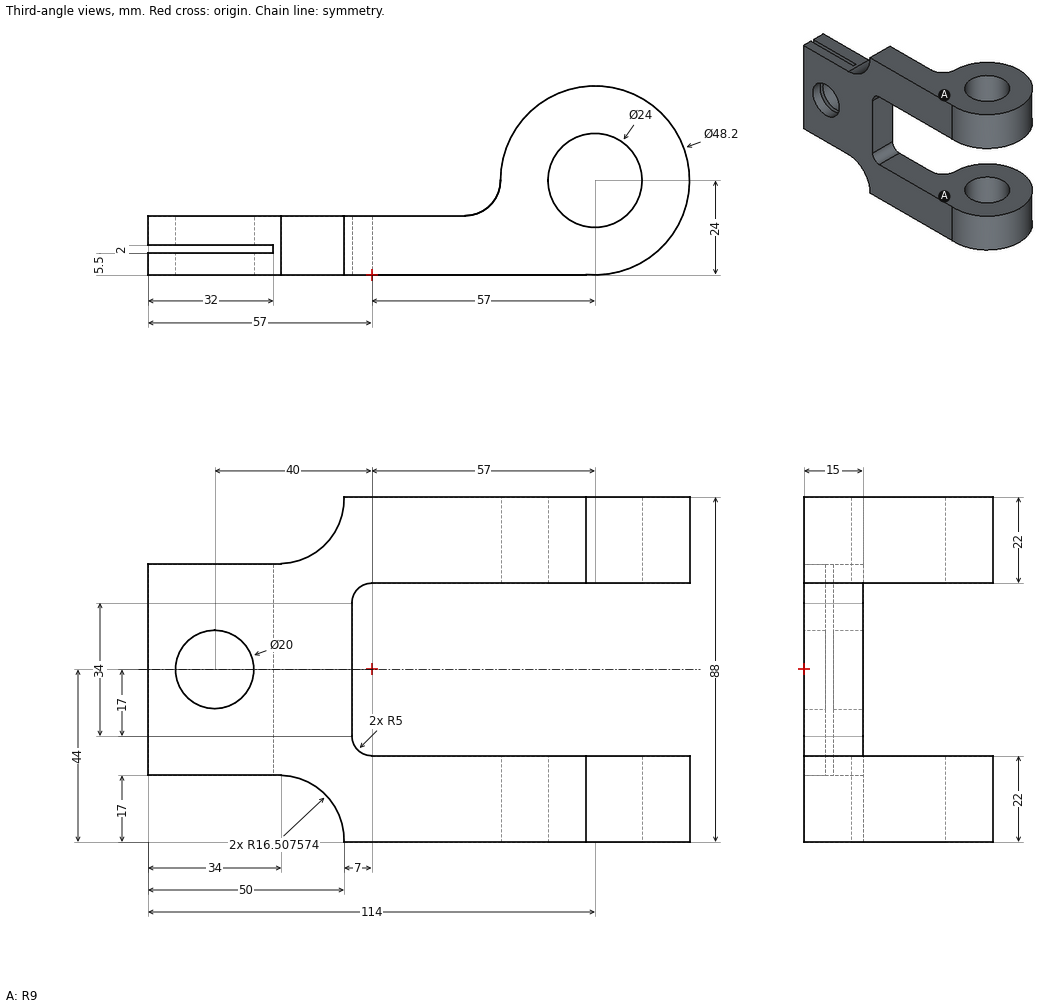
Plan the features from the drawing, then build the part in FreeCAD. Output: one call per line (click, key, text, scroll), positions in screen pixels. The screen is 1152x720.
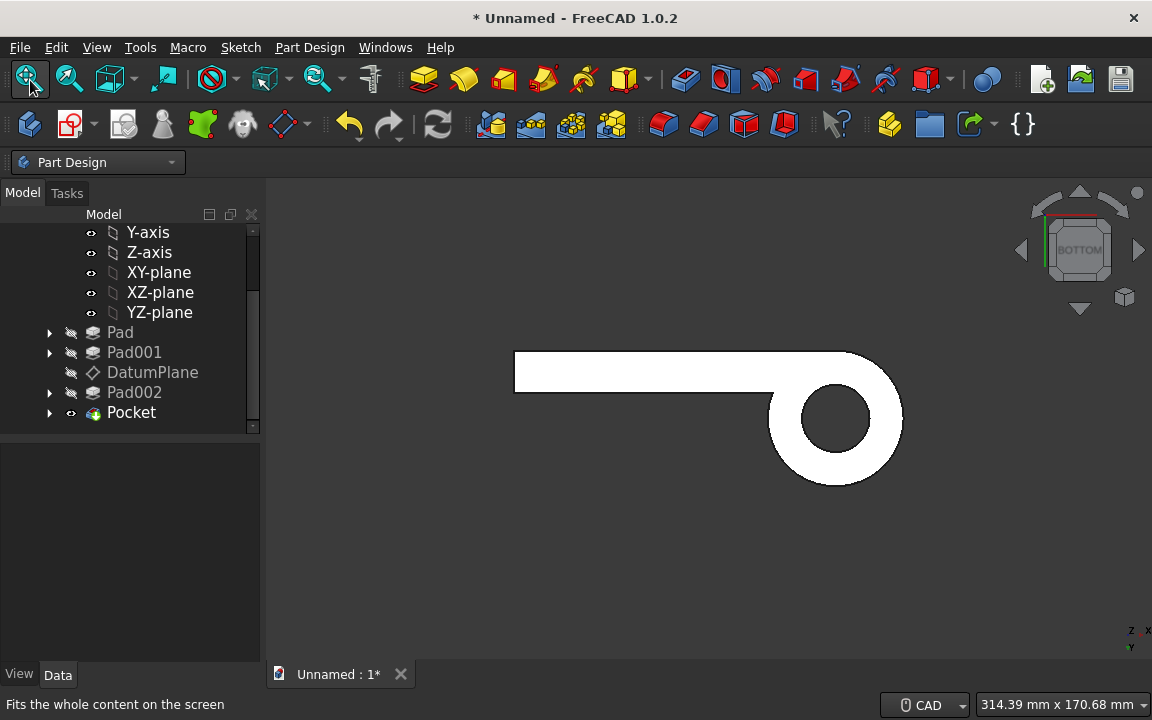
key(4)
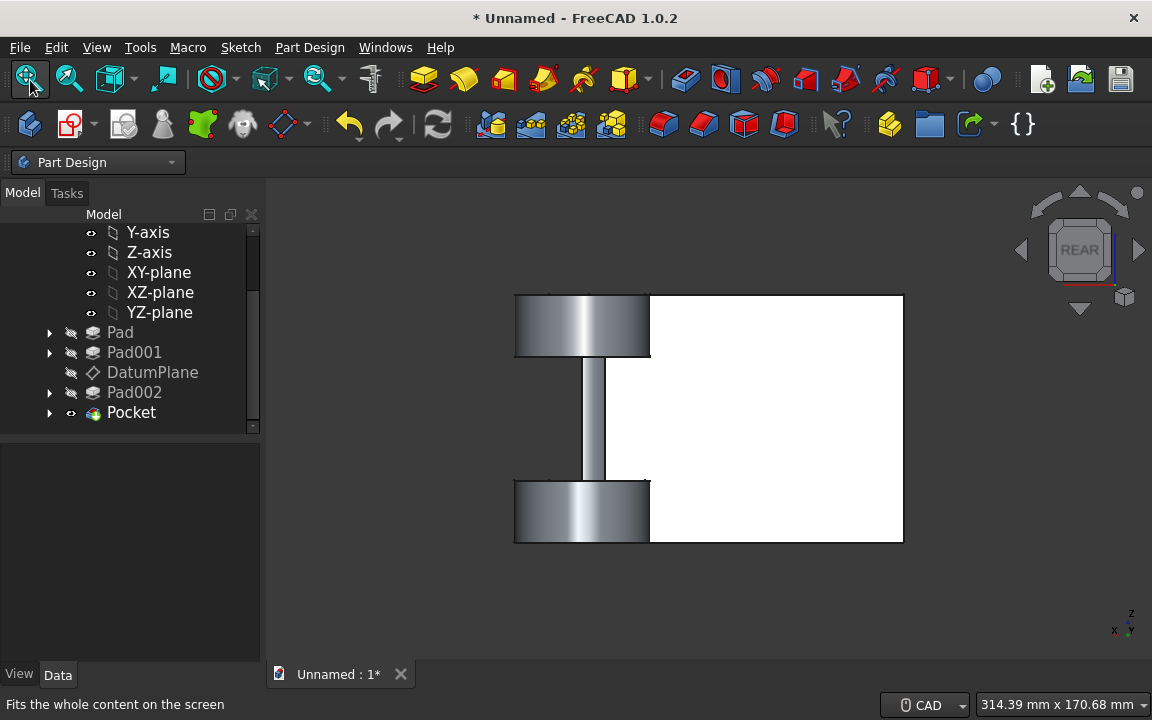
key(6)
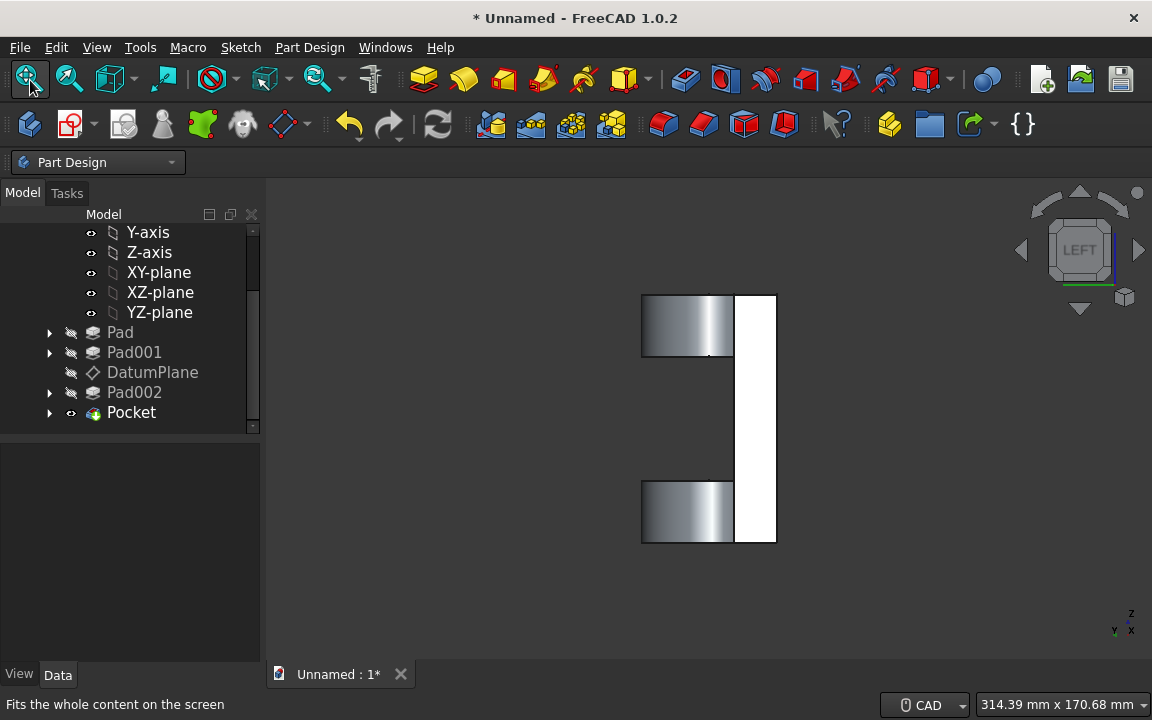
key(v)
key(3)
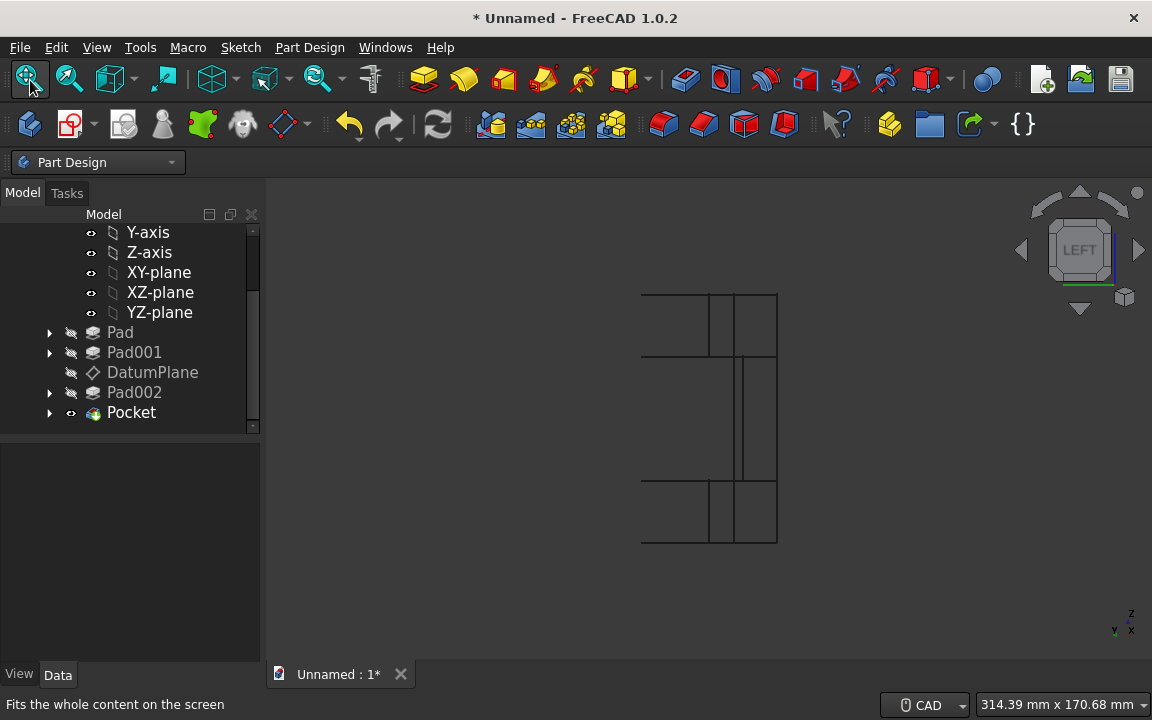
key(0)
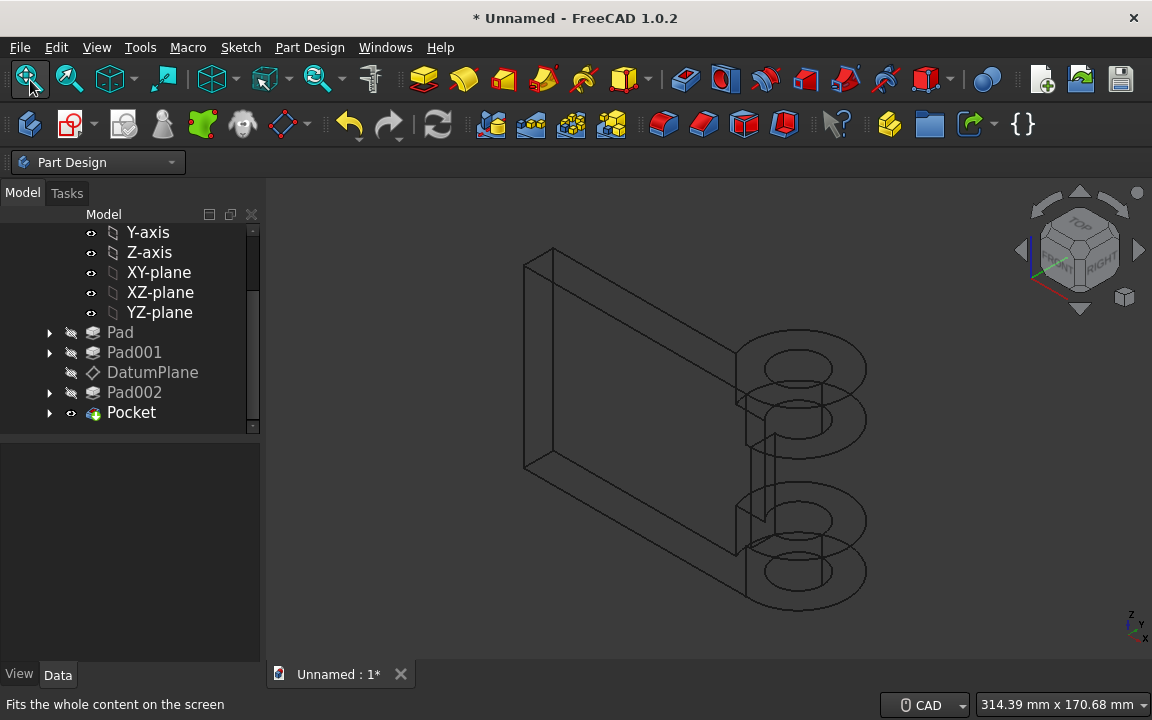
click(736, 378)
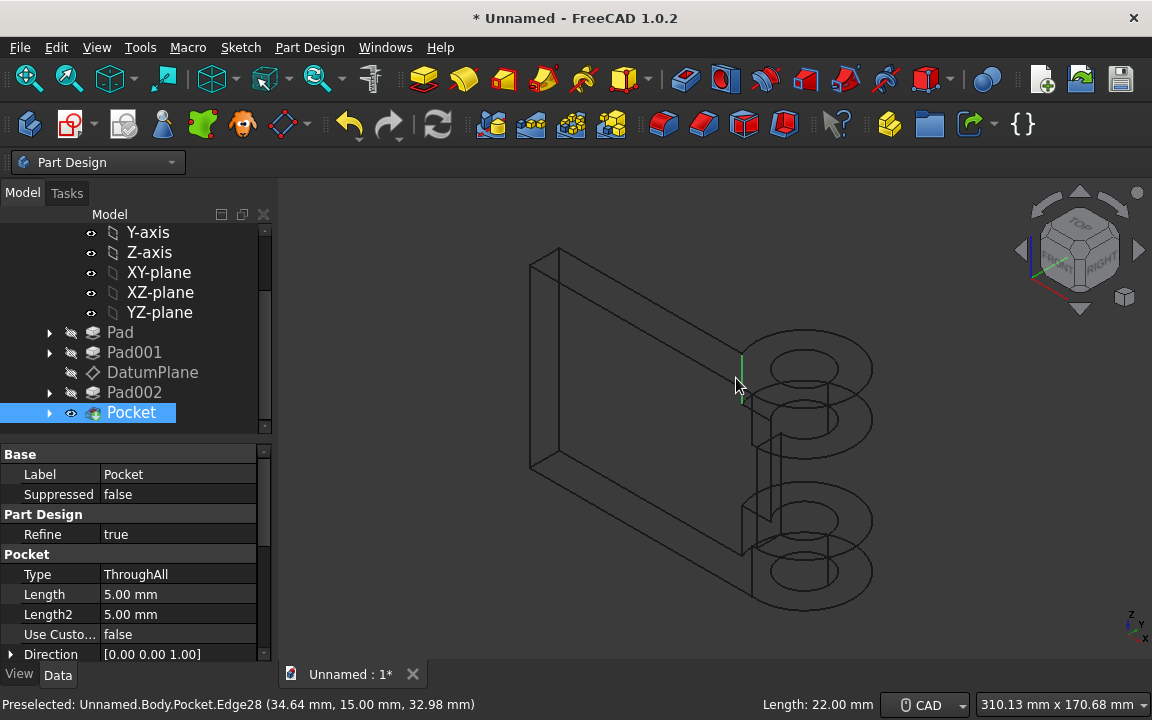
click(742, 530, ctrl)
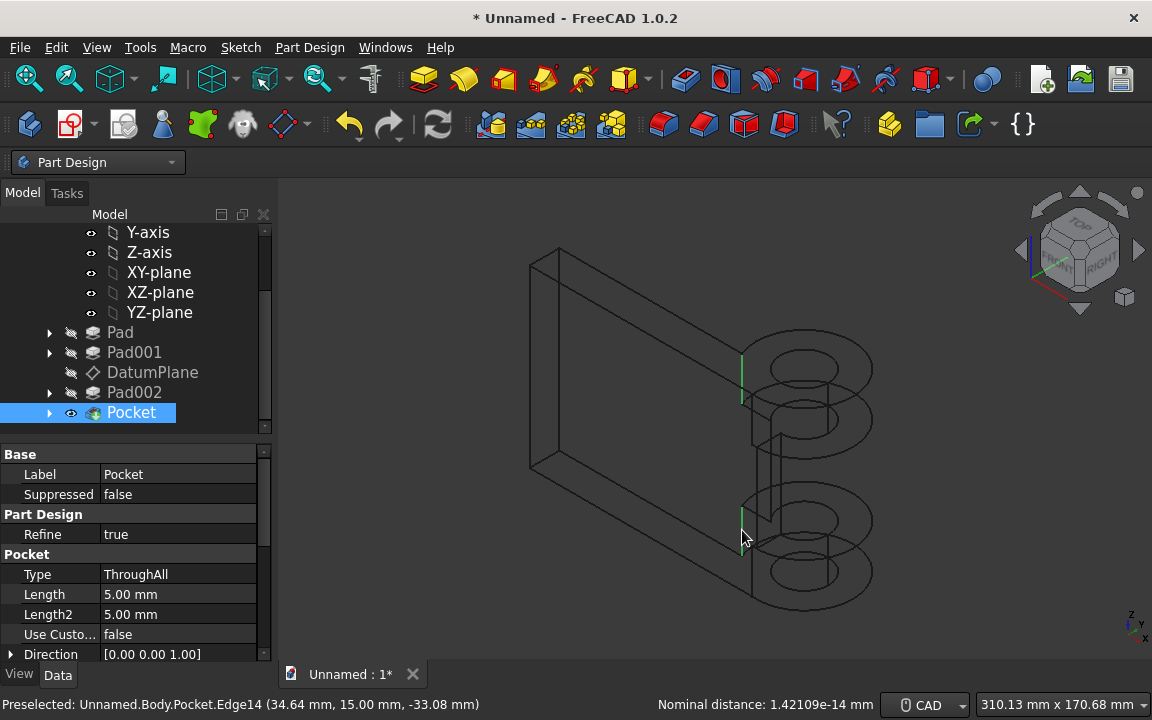
key(v)
key(1)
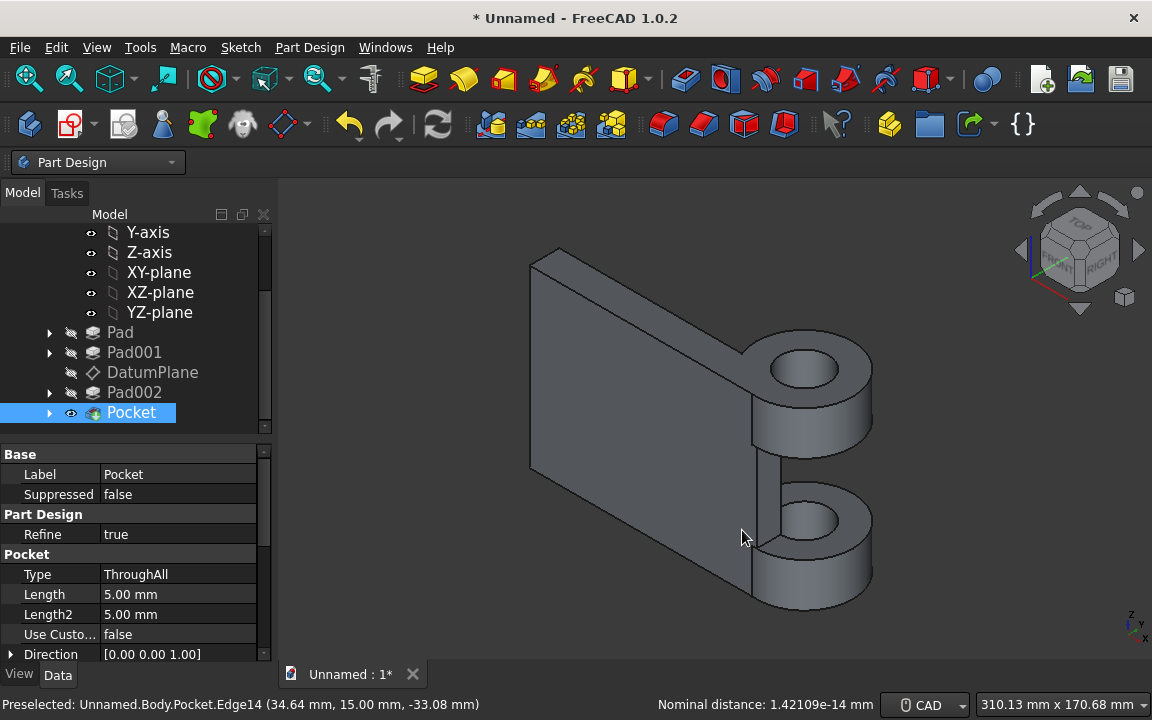
click(664, 124)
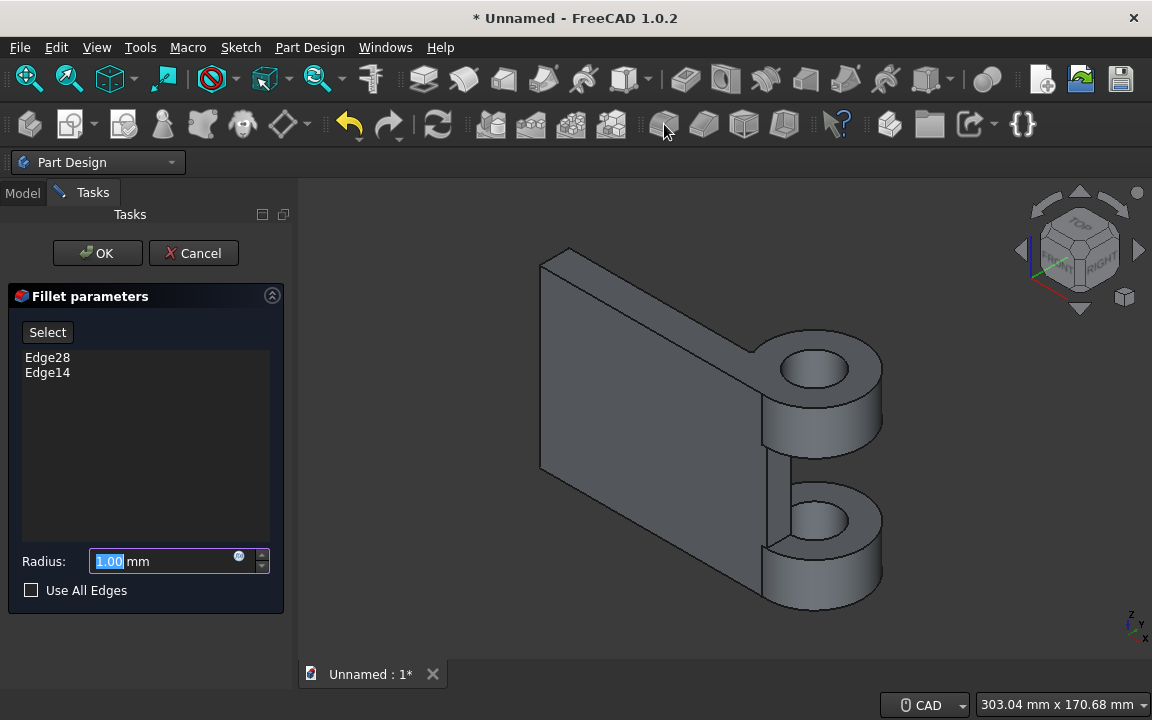
text(9)
key(Tab)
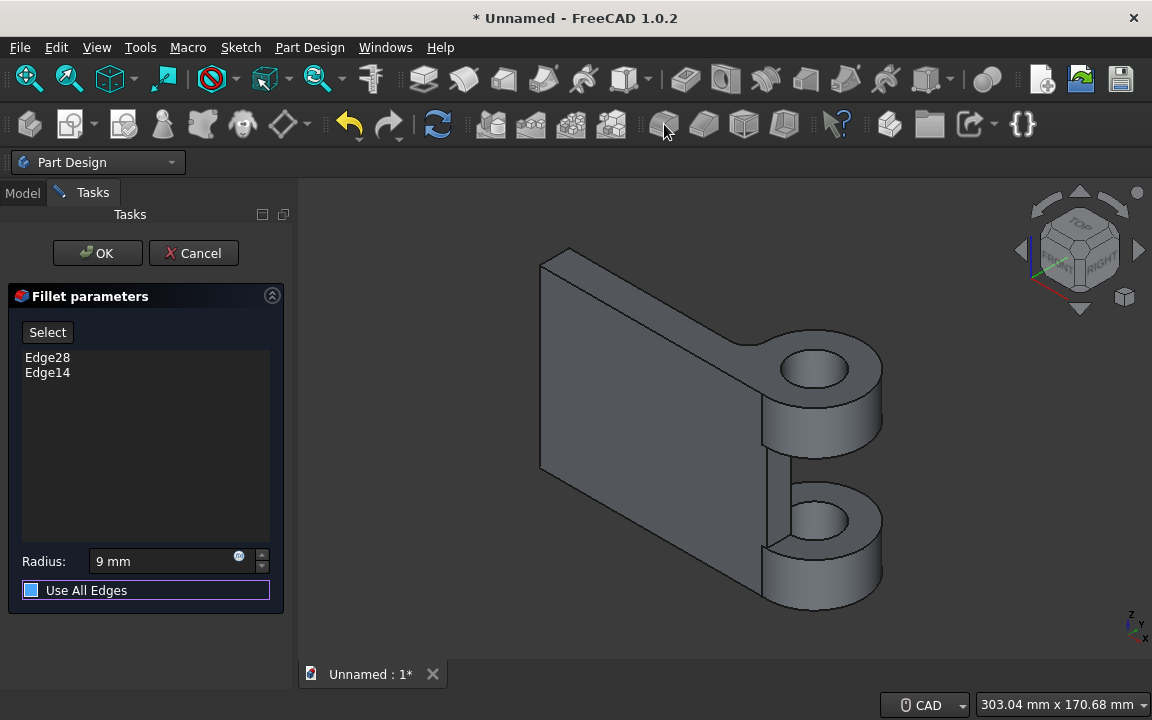
click(98, 253)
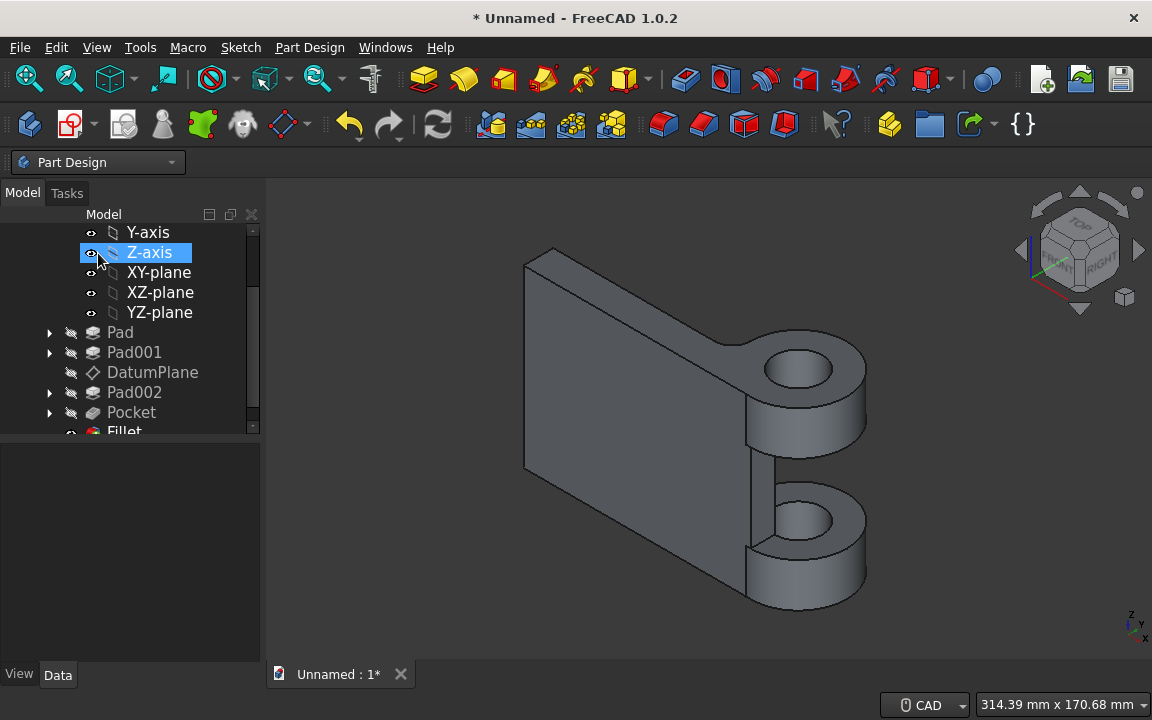
key(4)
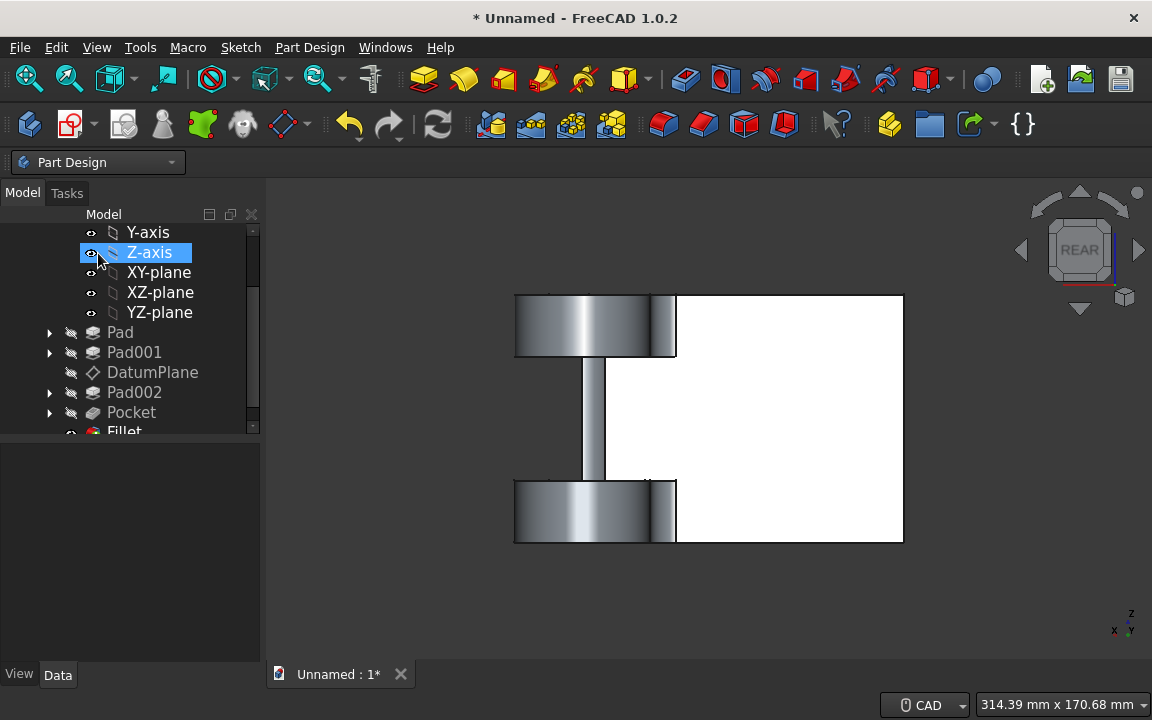
click(797, 417)